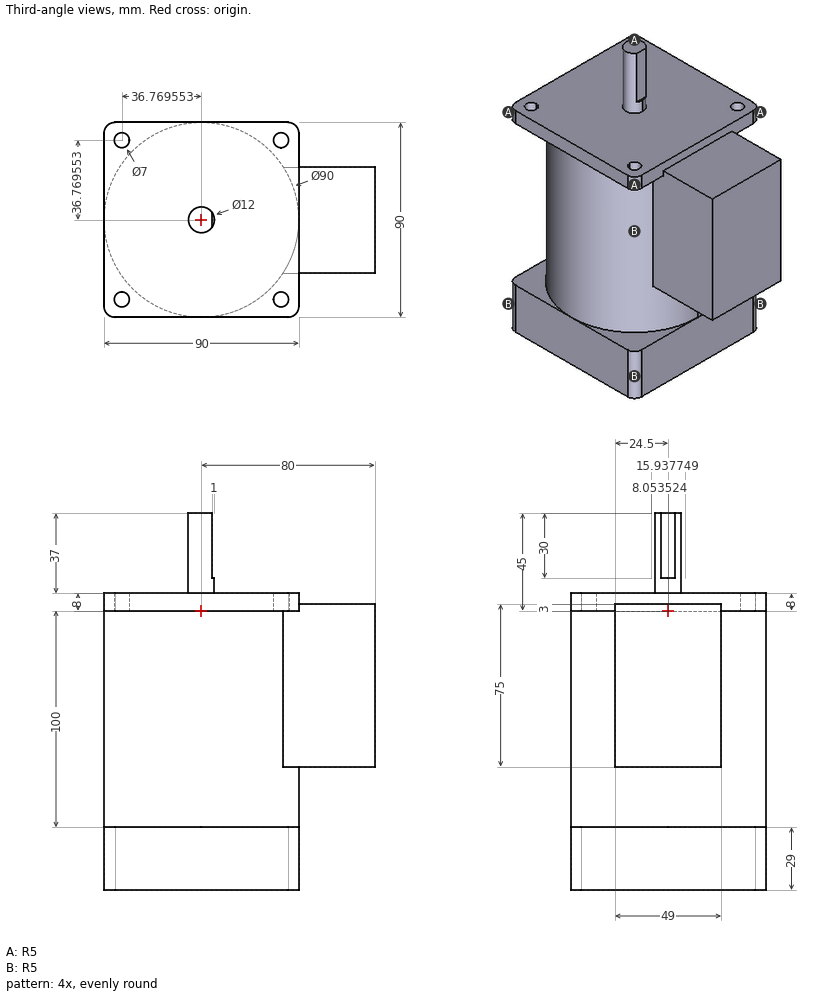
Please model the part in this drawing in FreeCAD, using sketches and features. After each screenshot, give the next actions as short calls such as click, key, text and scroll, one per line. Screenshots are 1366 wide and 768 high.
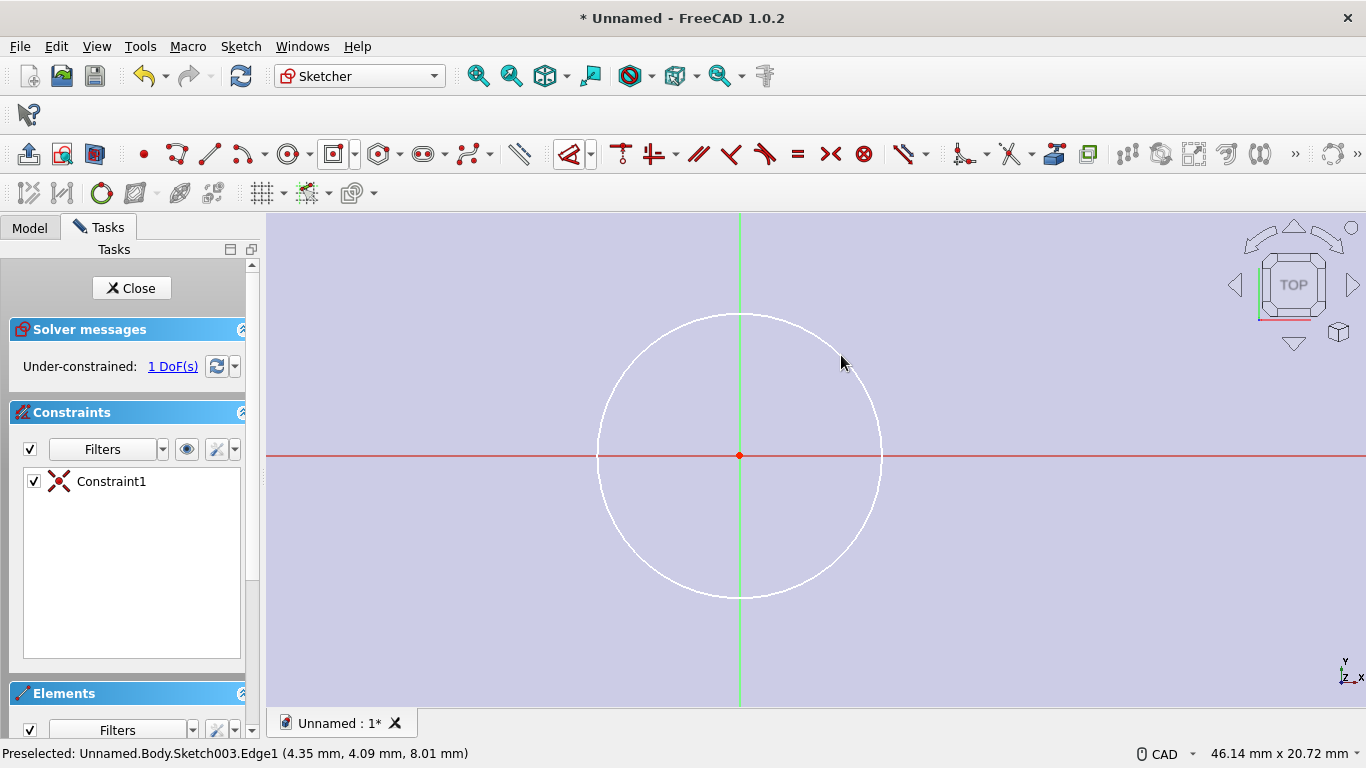
click(840, 355)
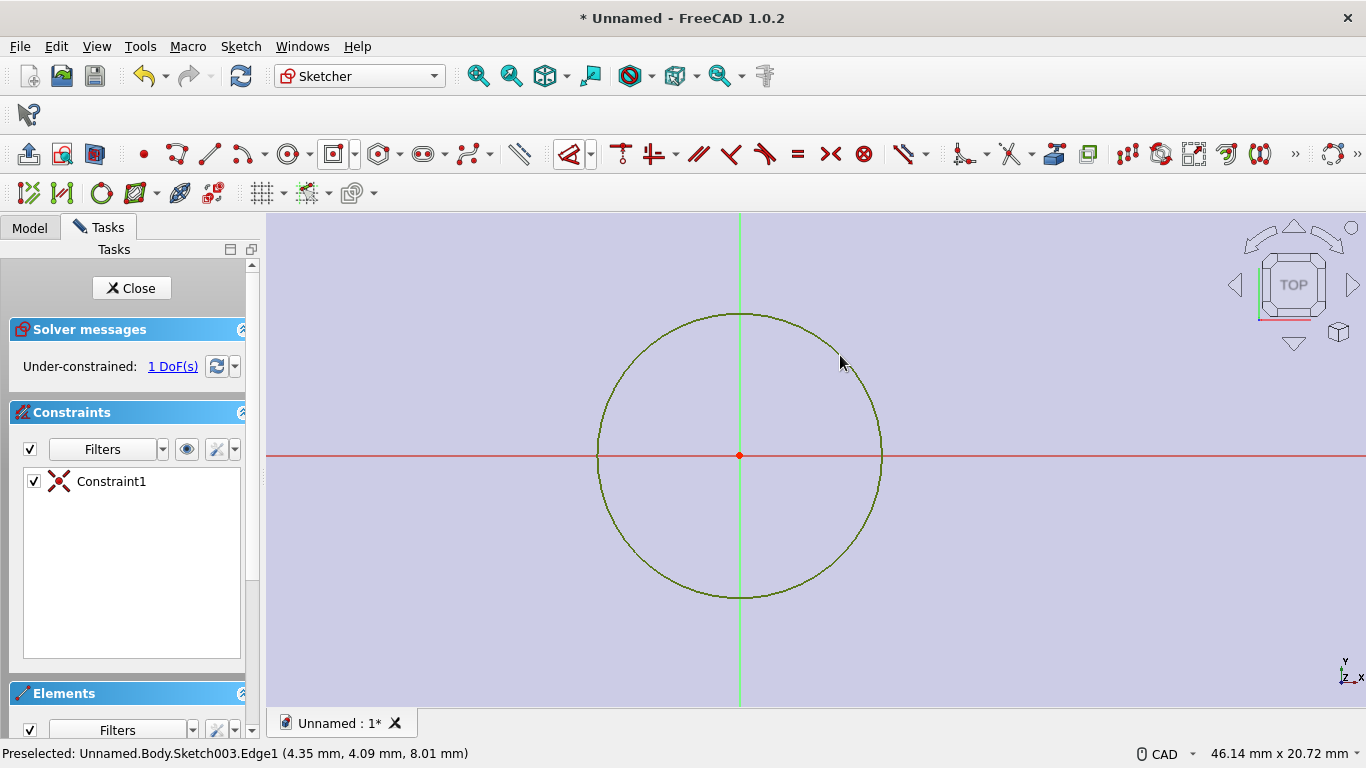
click(590, 154)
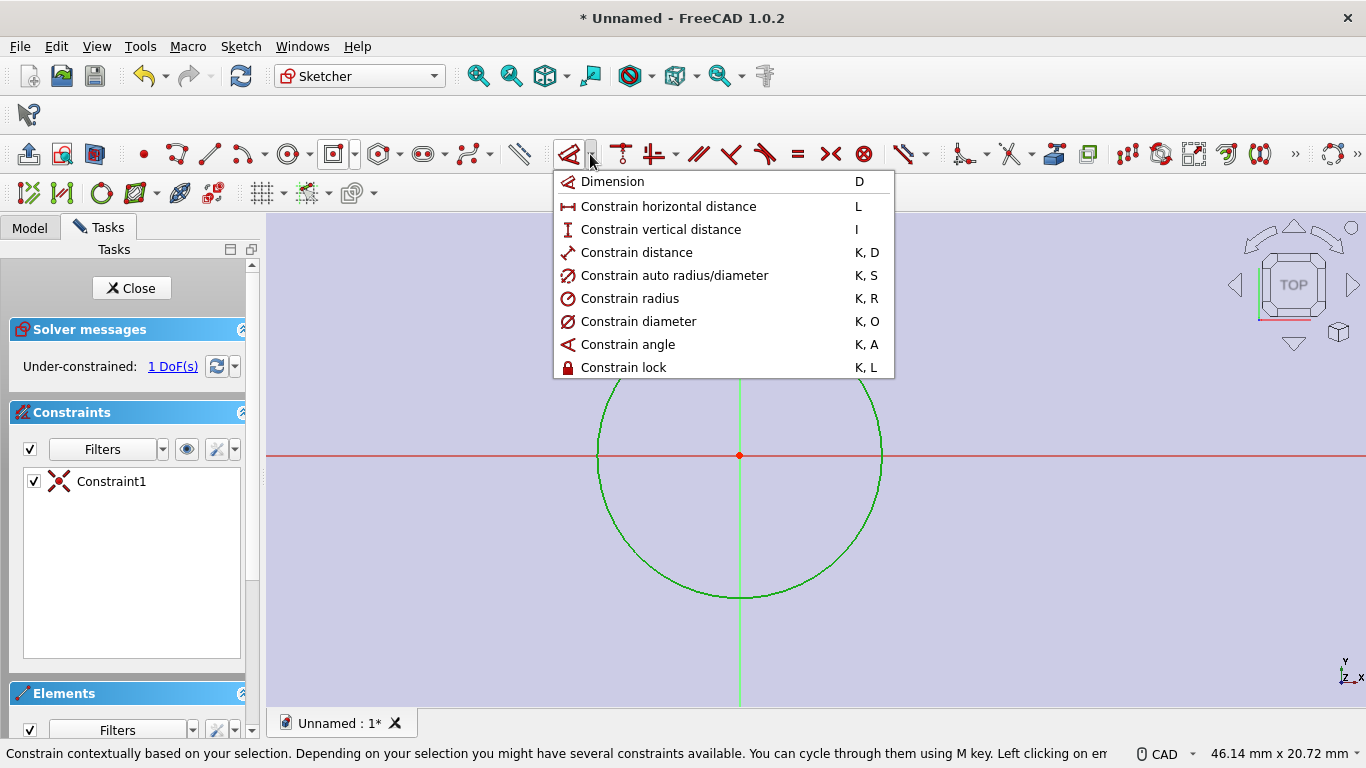
click(724, 322)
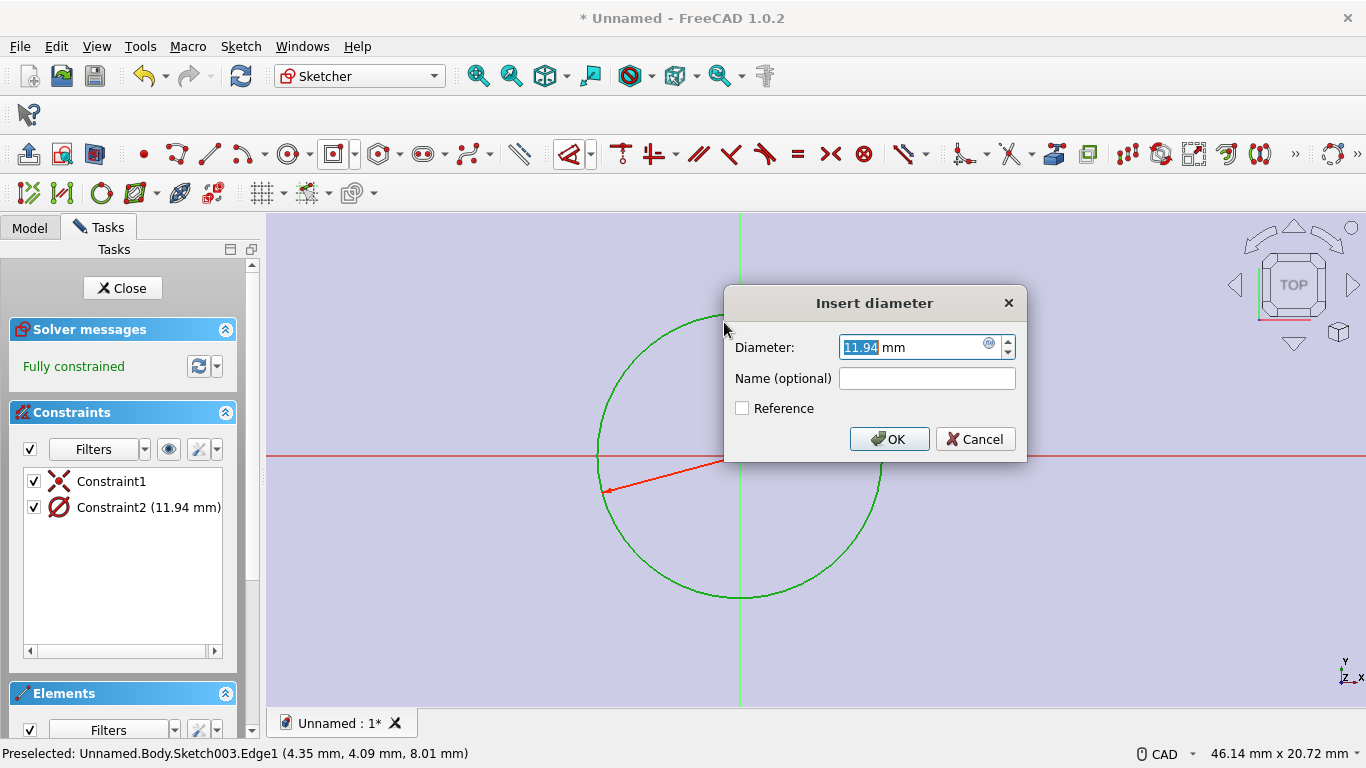
text(12)
key(Return)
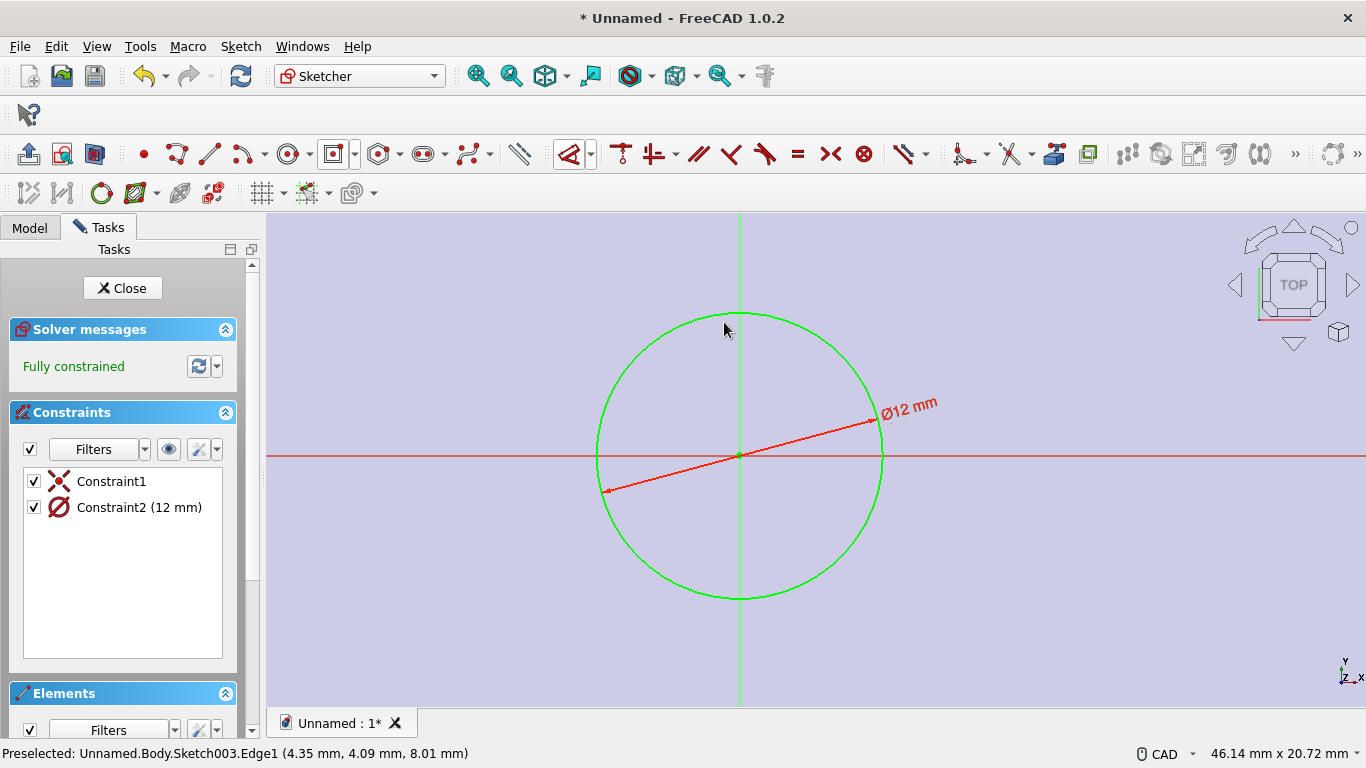
click(123, 288)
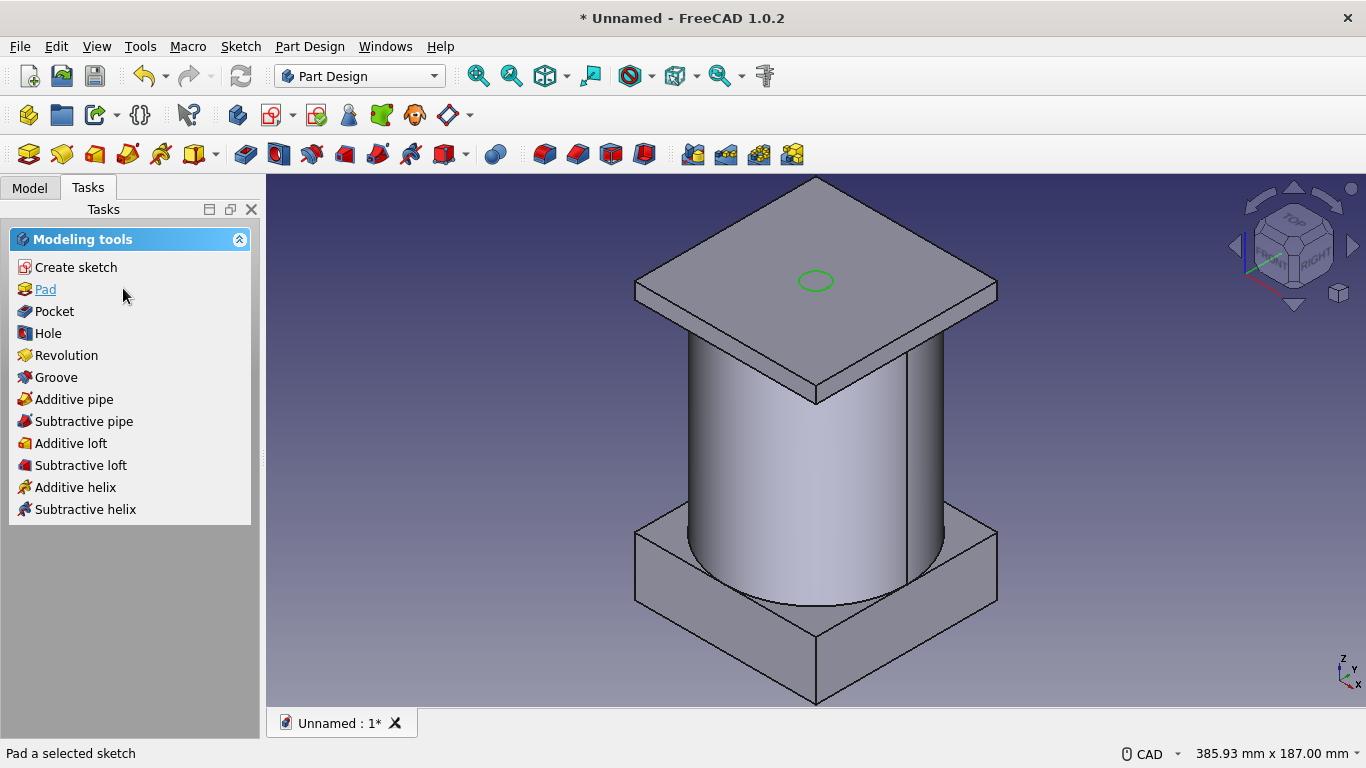
click(29, 154)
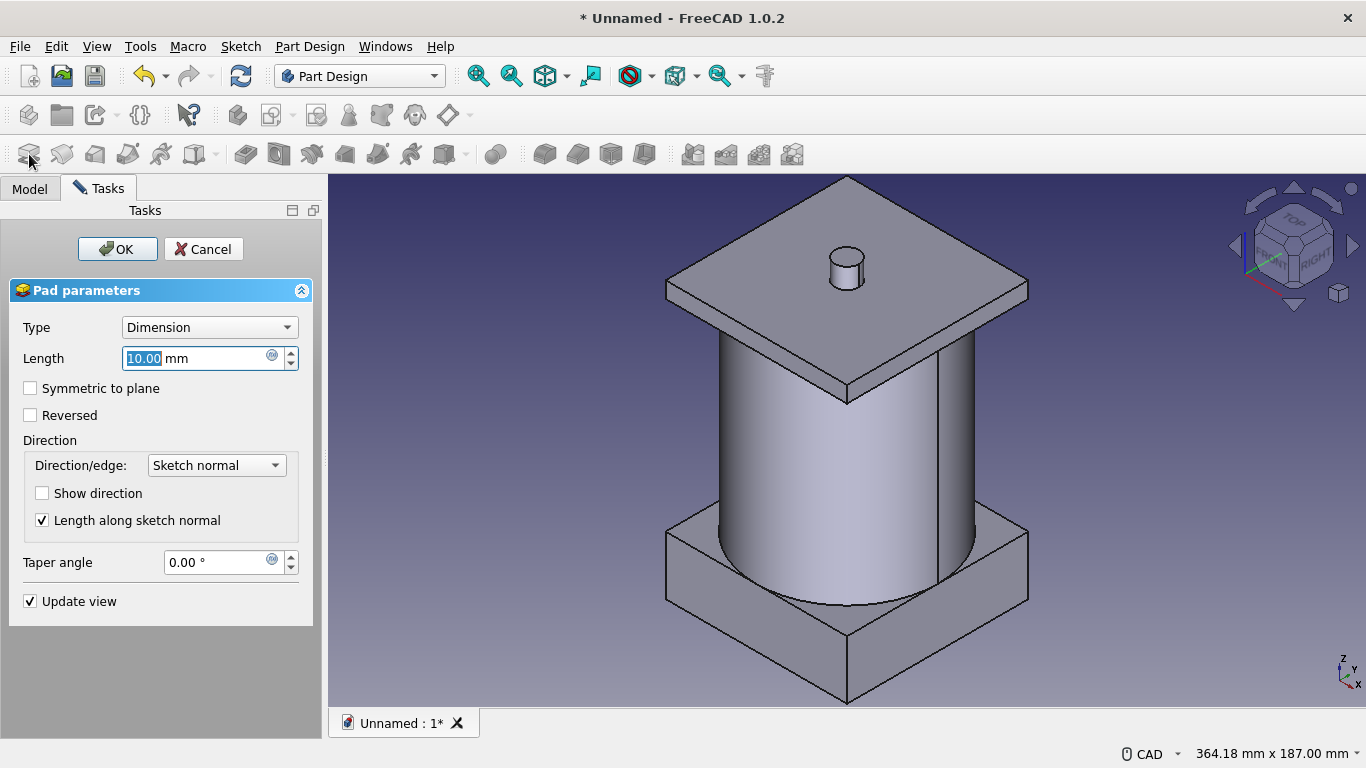
text(37)
key(Tab)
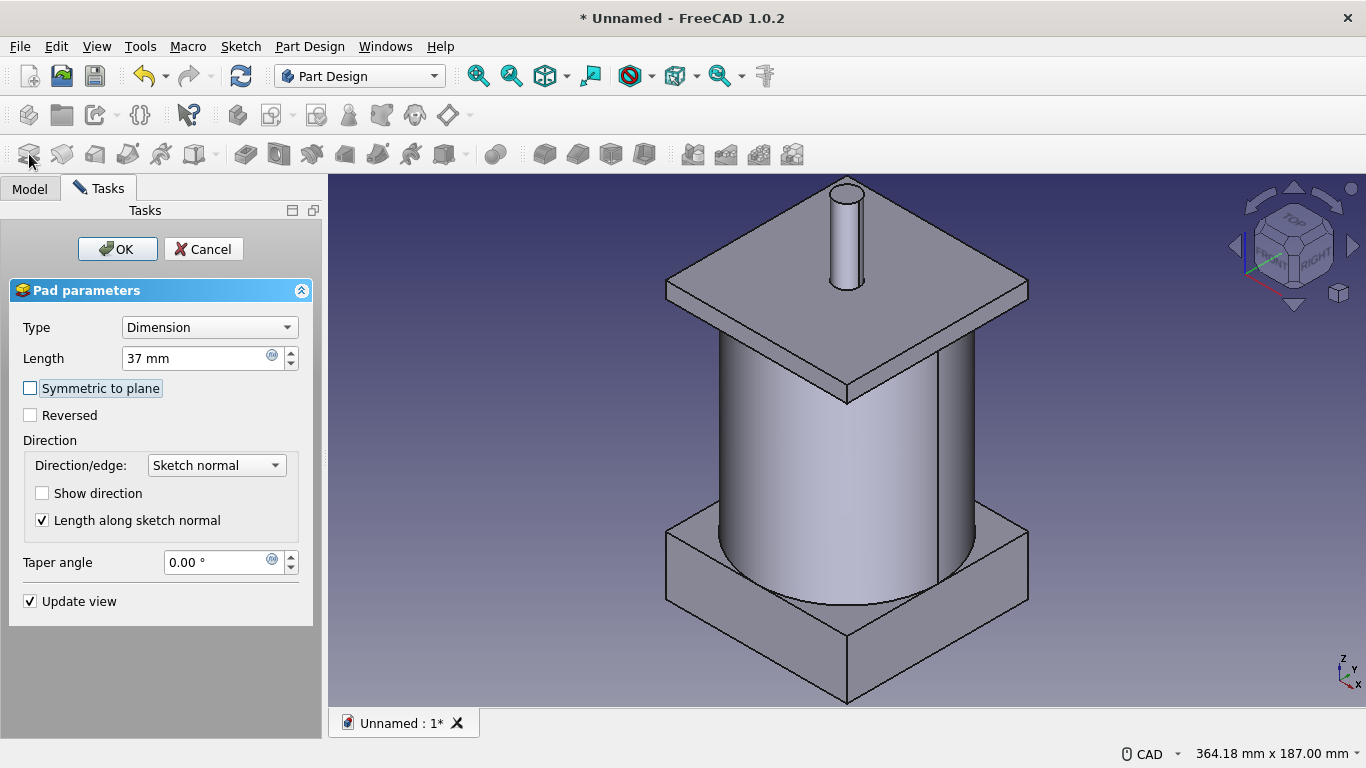
click(118, 249)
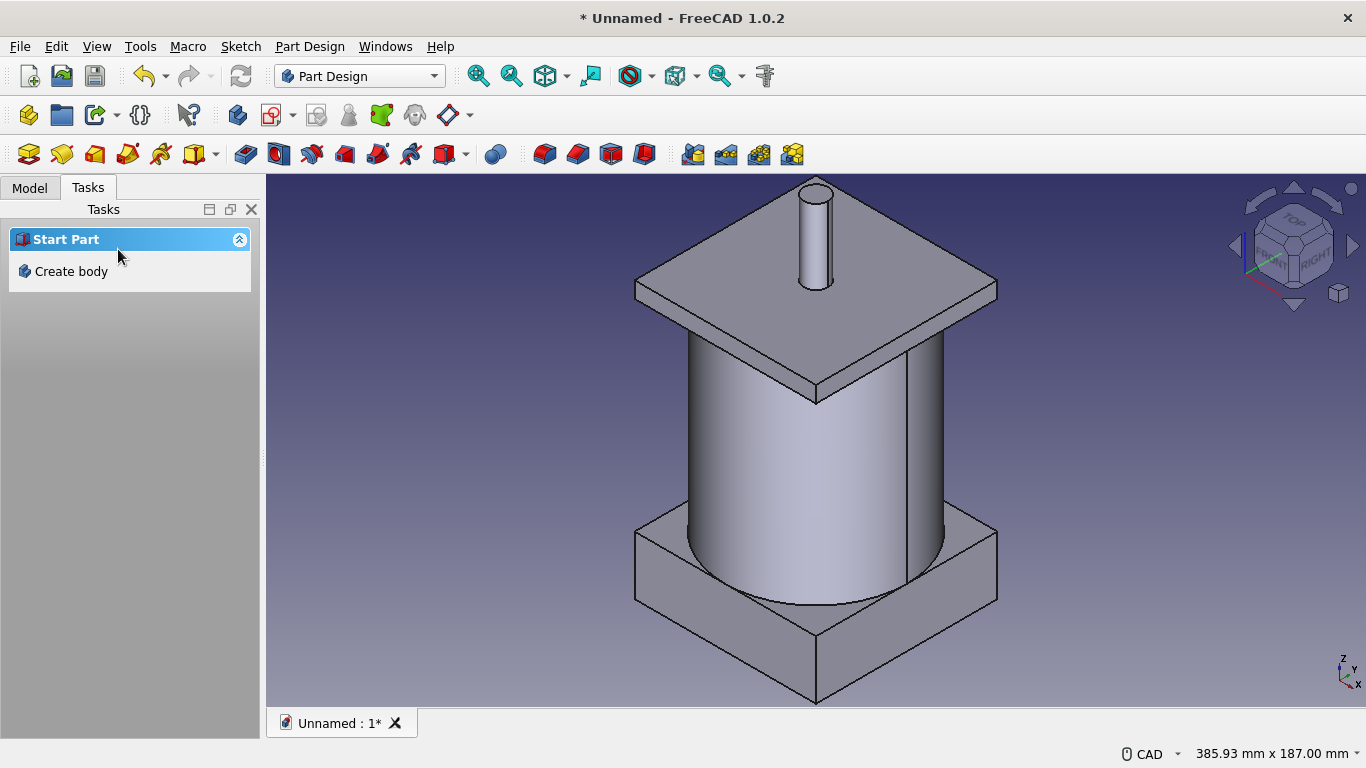
key(v)
key(f)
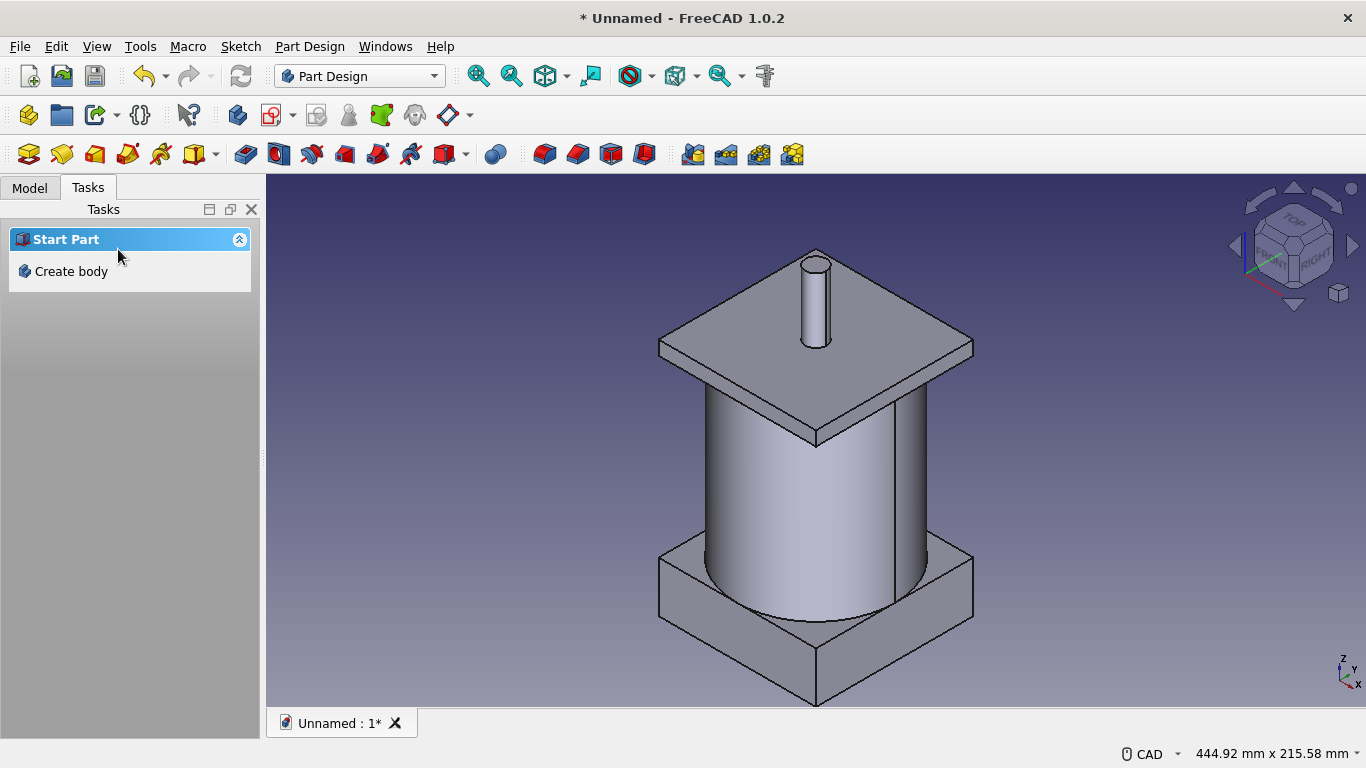
click(270, 116)